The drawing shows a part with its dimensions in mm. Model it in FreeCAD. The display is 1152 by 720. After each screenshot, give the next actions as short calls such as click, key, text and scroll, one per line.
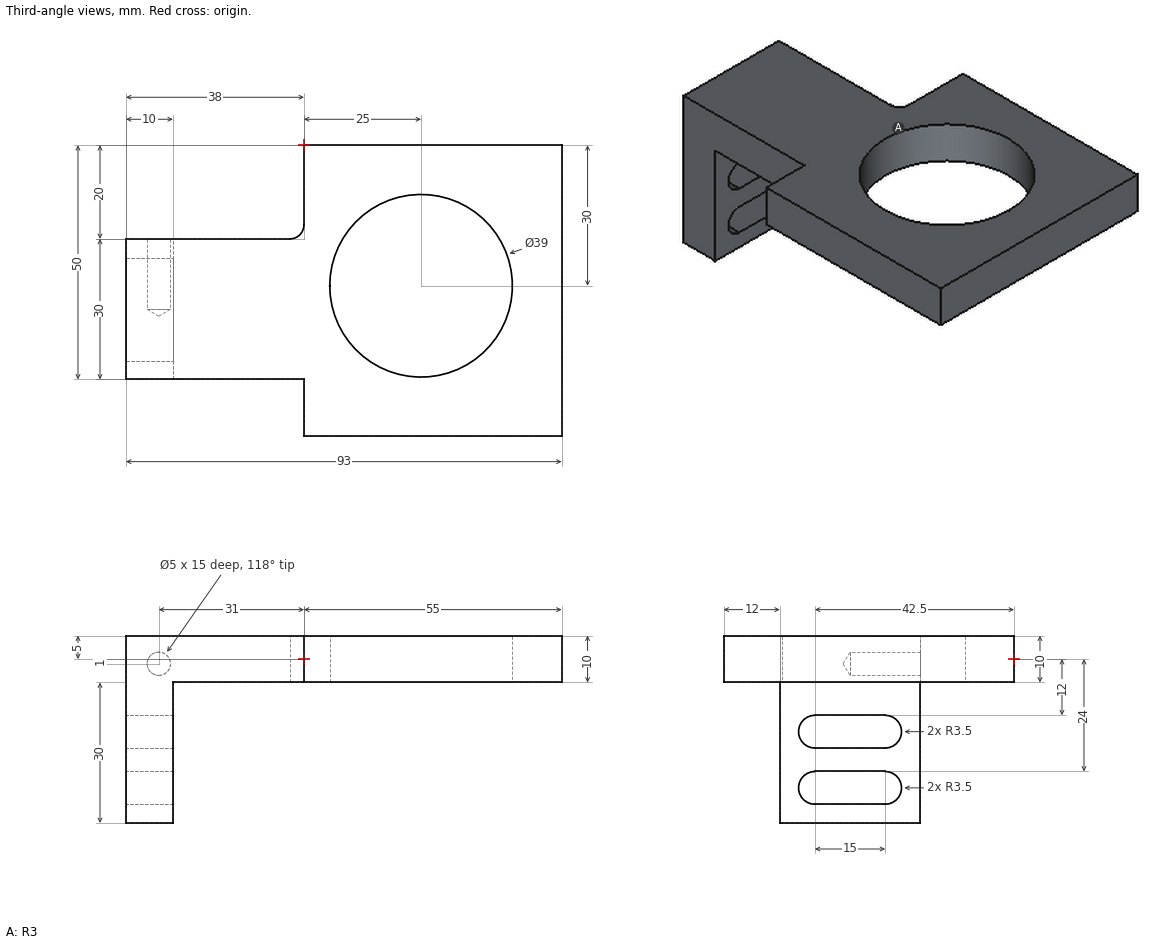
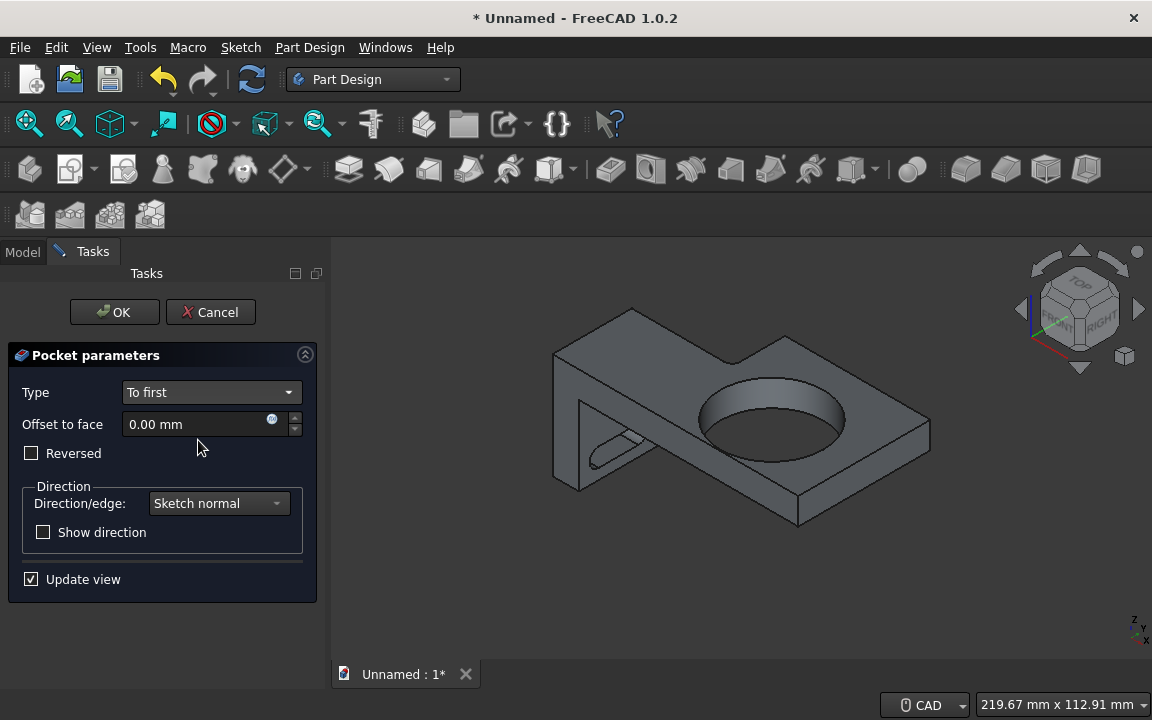
click(115, 312)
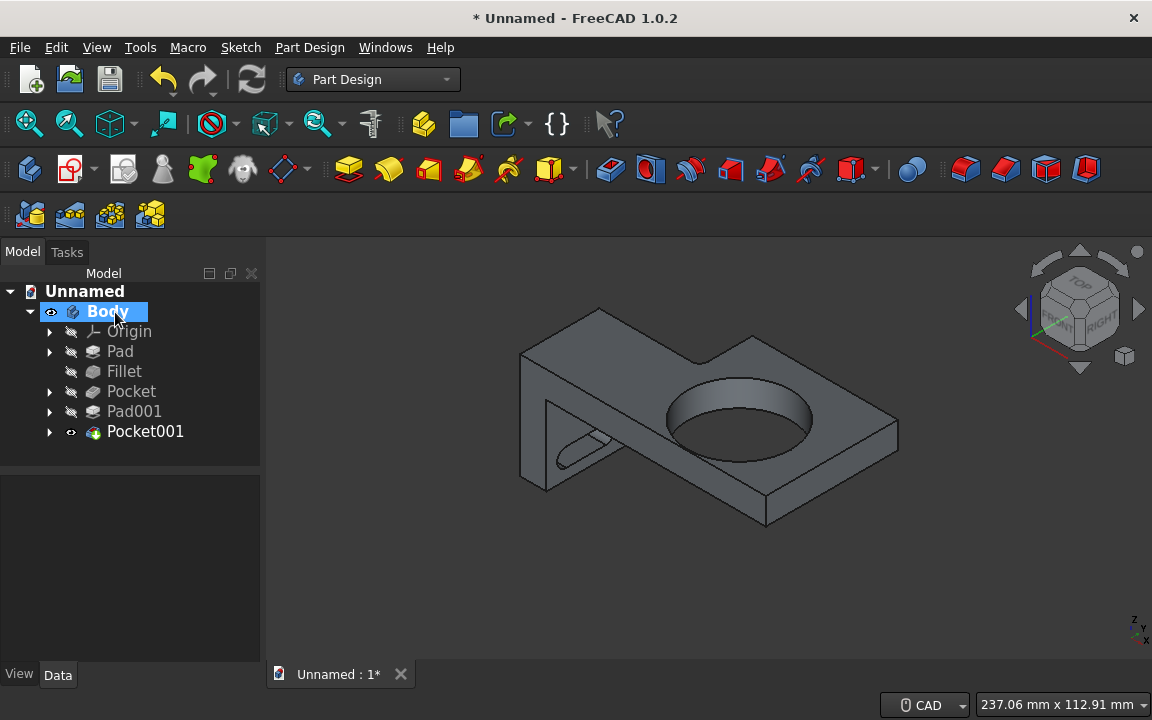
click(563, 422)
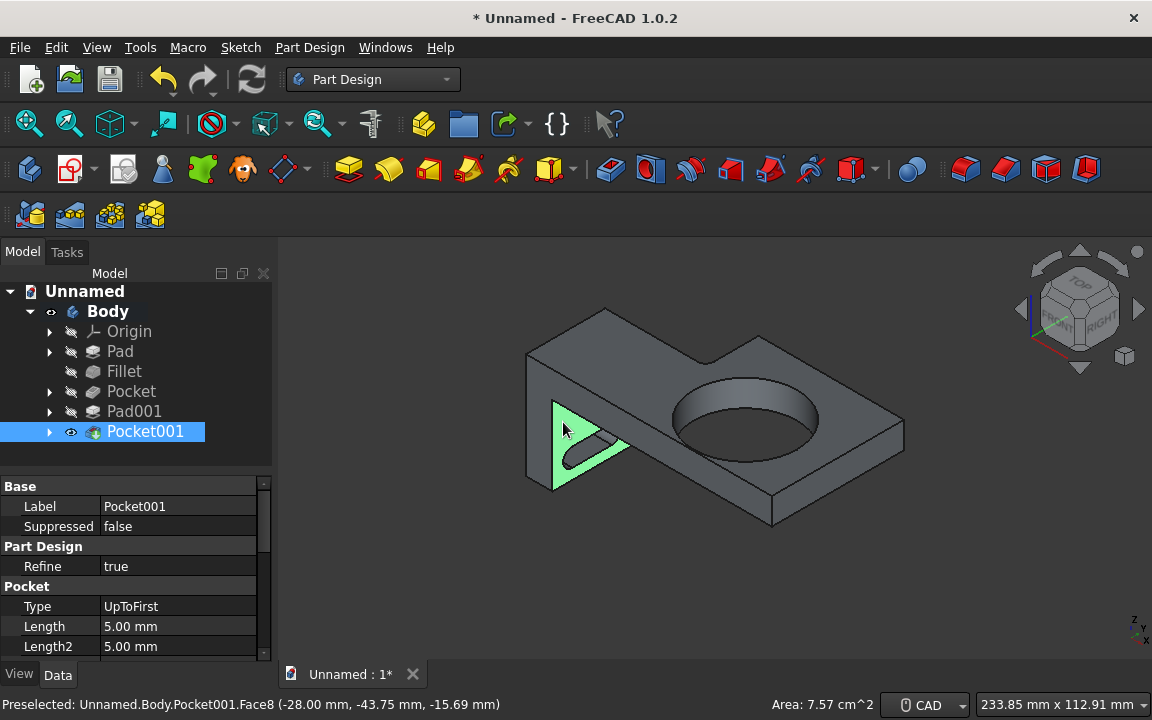
click(70, 170)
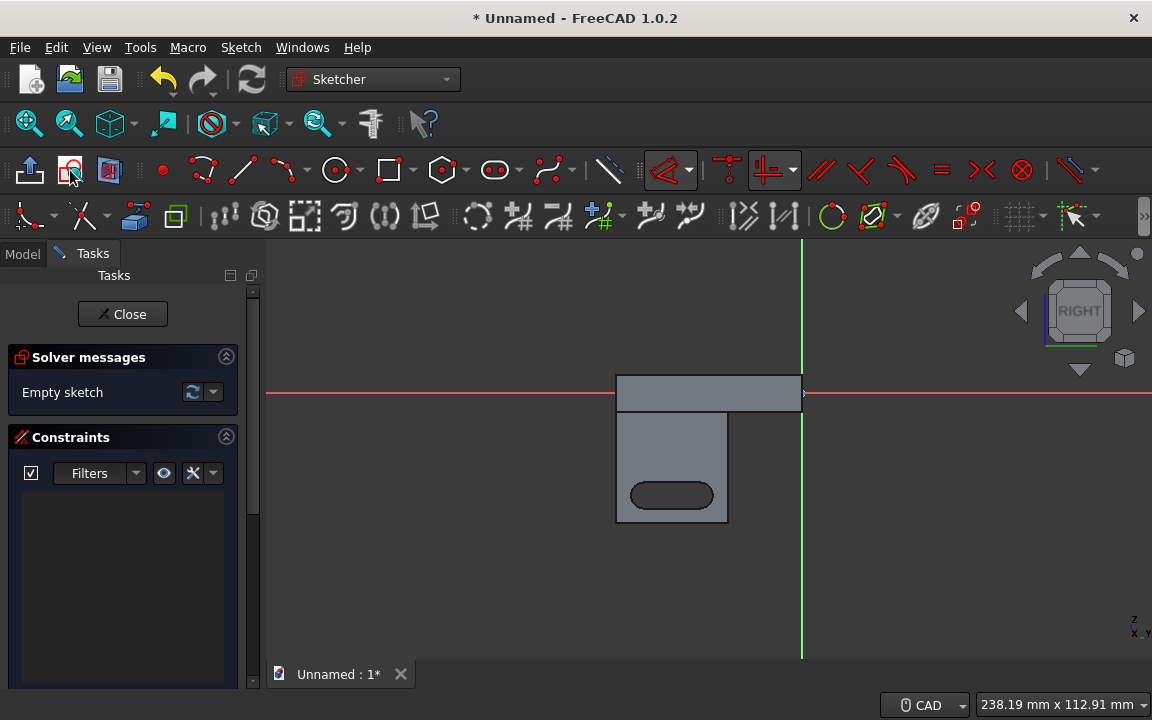
key(q)
key(s)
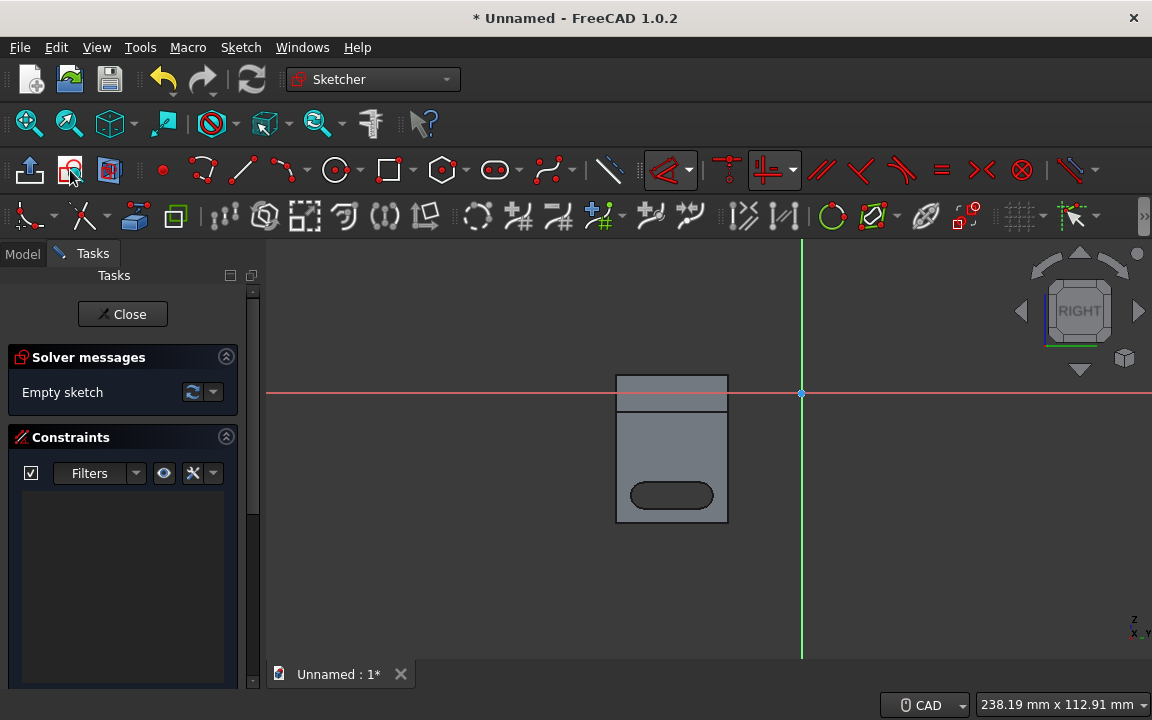
scroll(761, 417, up, 5)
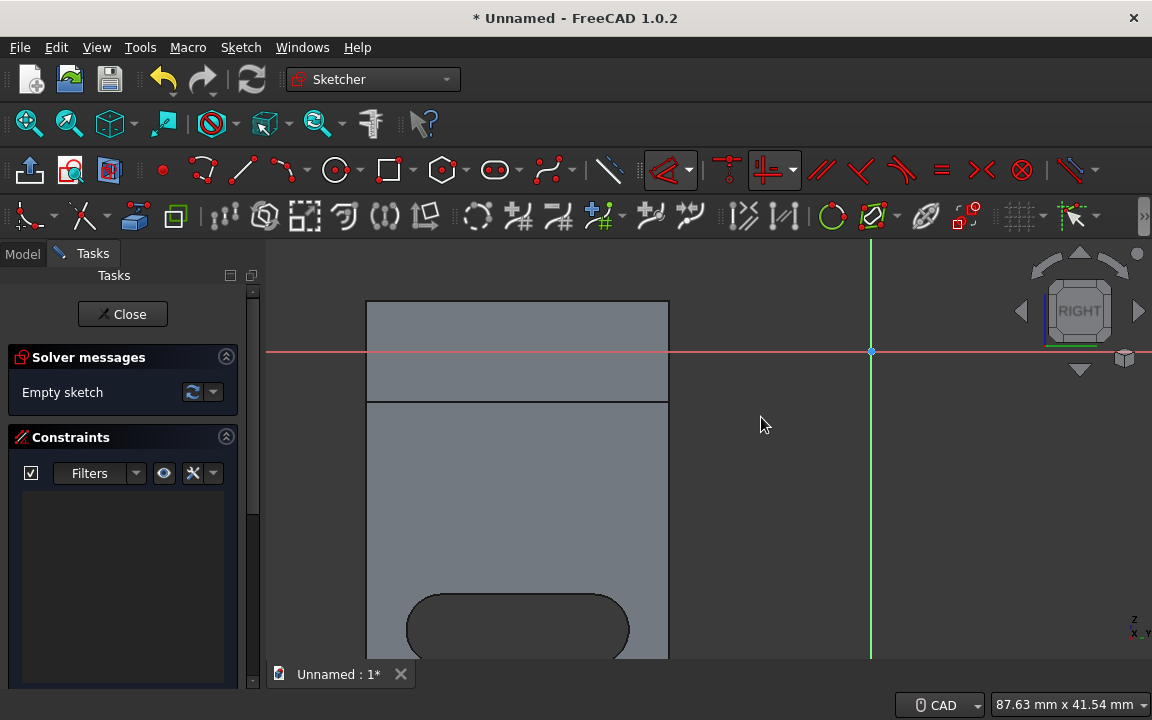
key(g)
key(s)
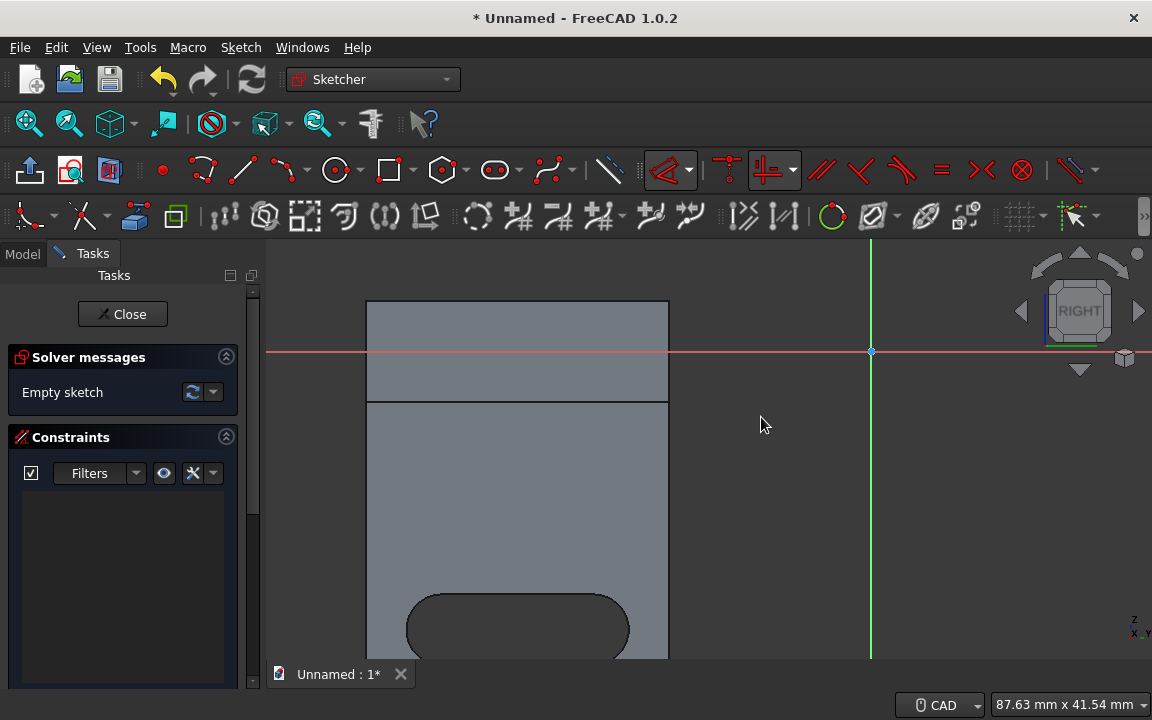
click(442, 508)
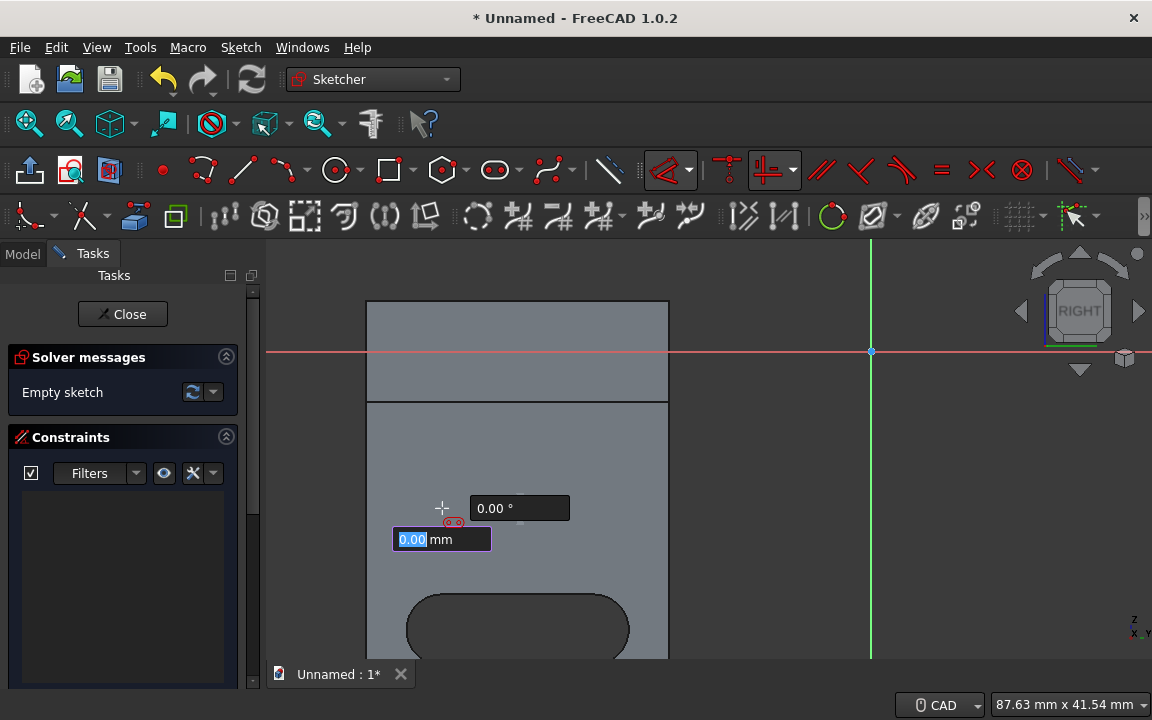
click(593, 508)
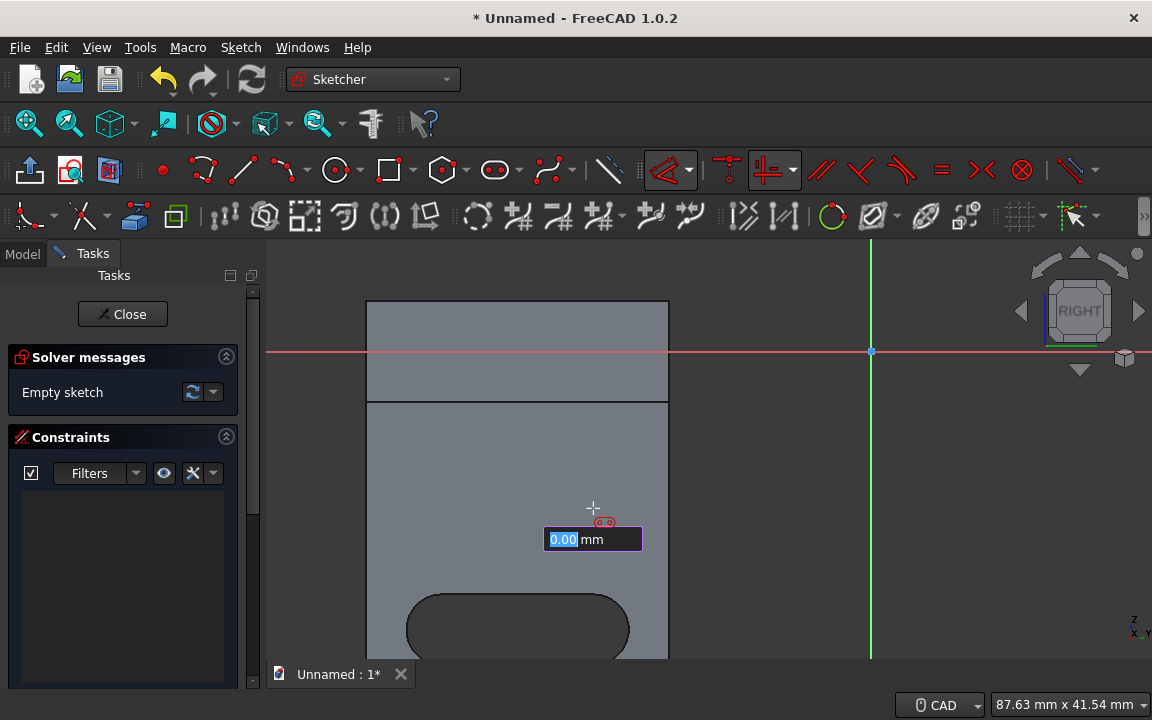
click(518, 544)
key(Escape)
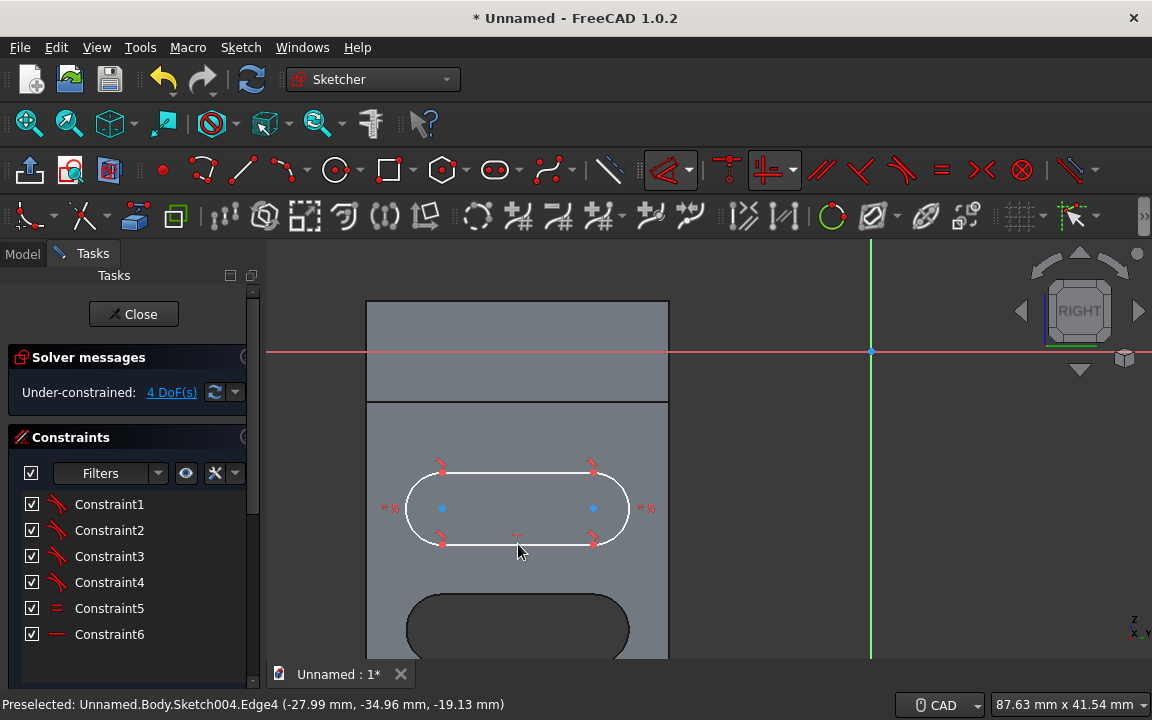
click(413, 488)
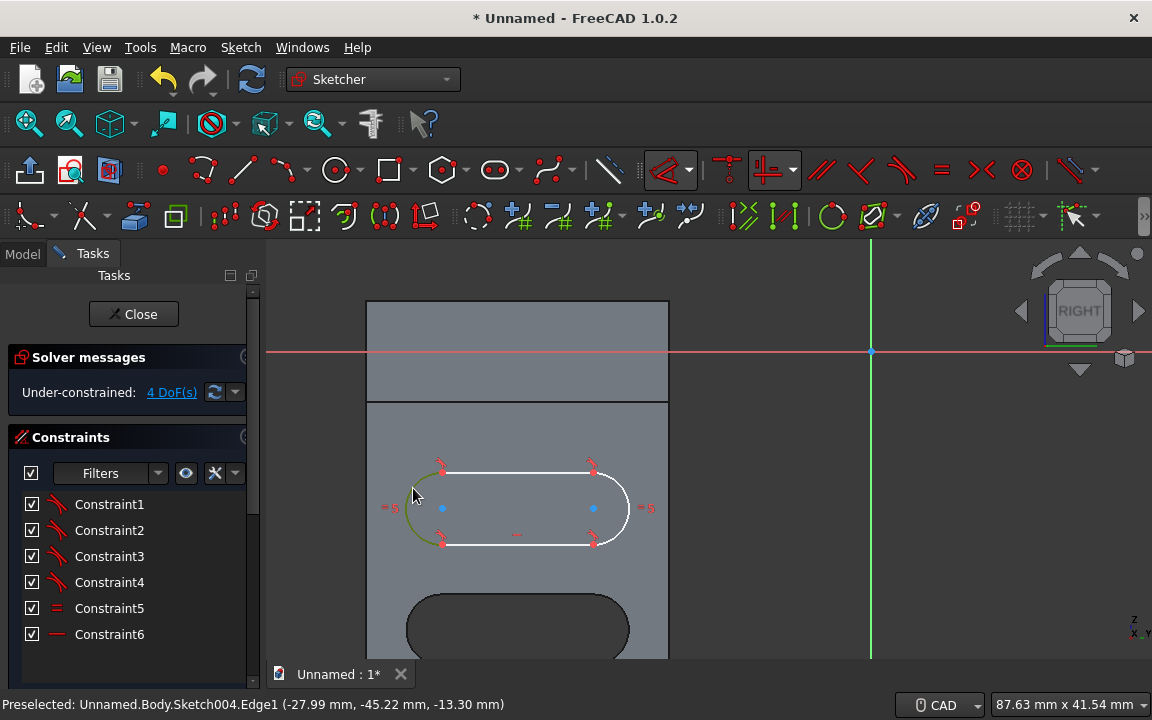
key(k)
key(r)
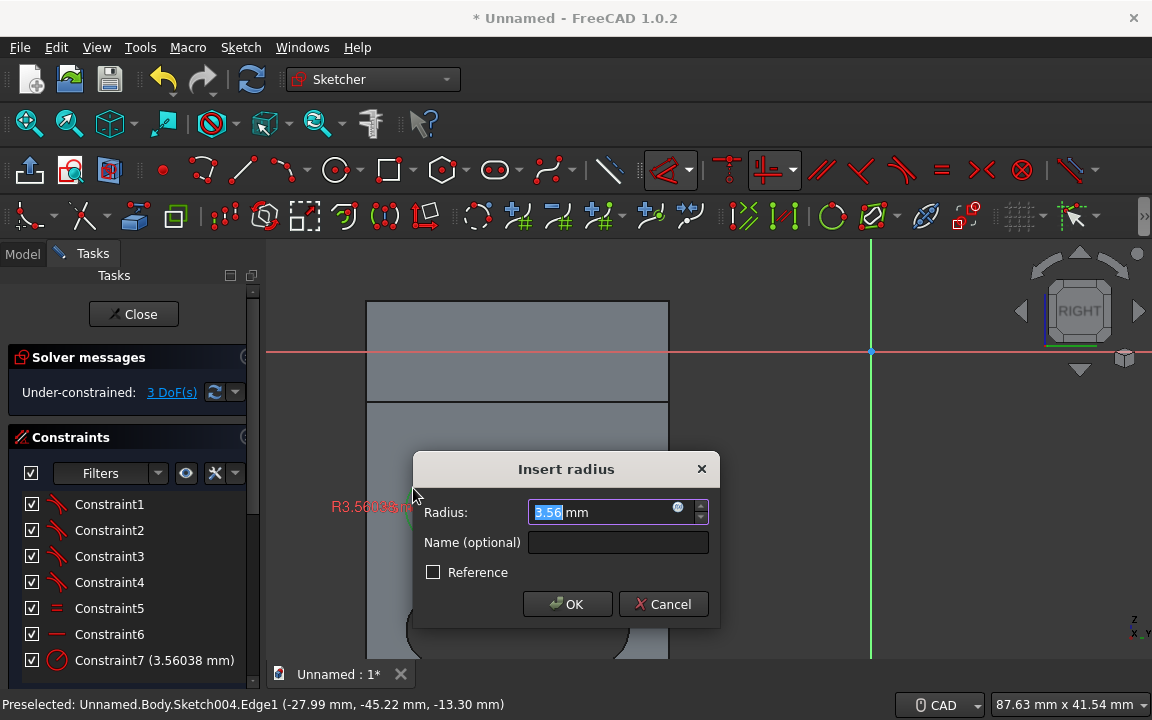
text(3.5)
key(Return)